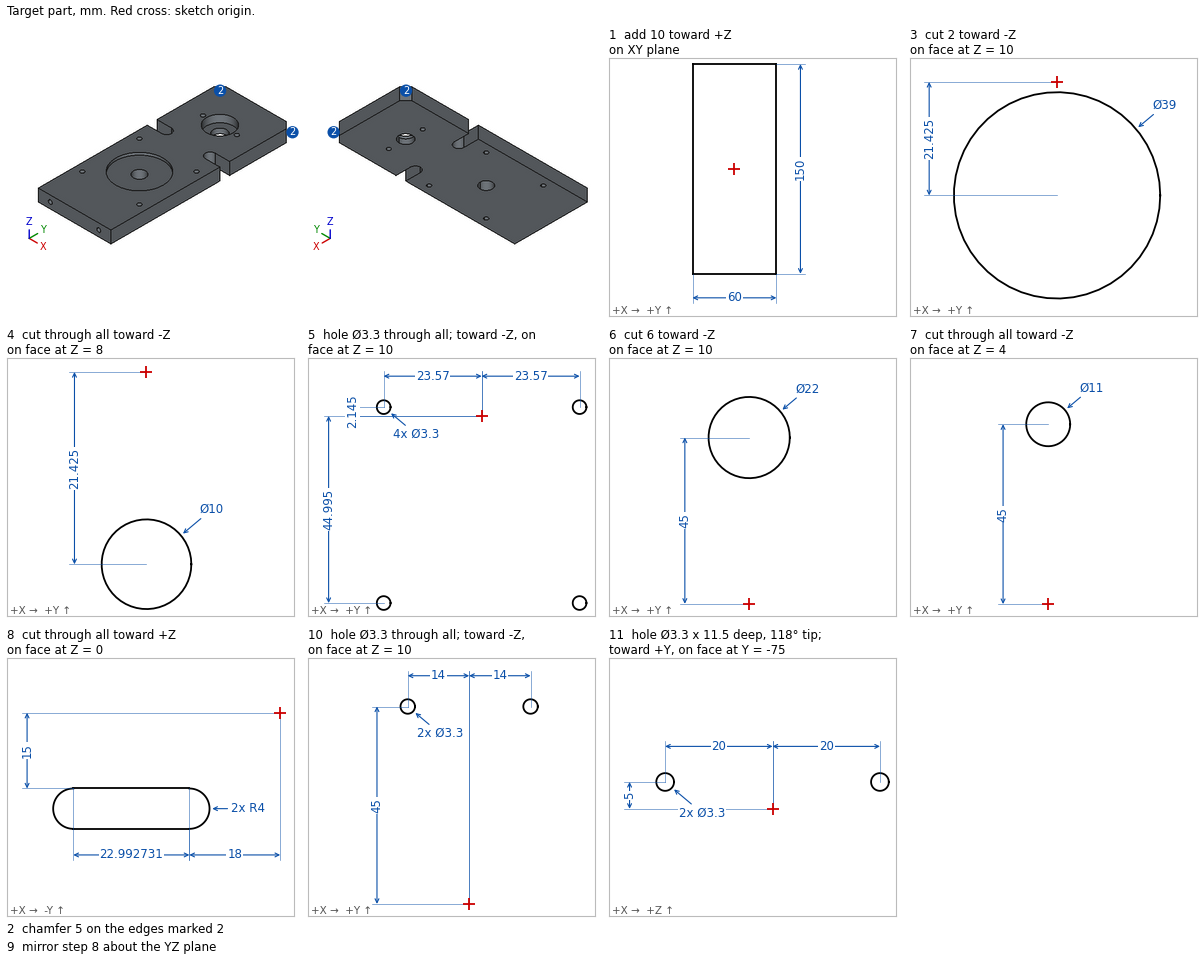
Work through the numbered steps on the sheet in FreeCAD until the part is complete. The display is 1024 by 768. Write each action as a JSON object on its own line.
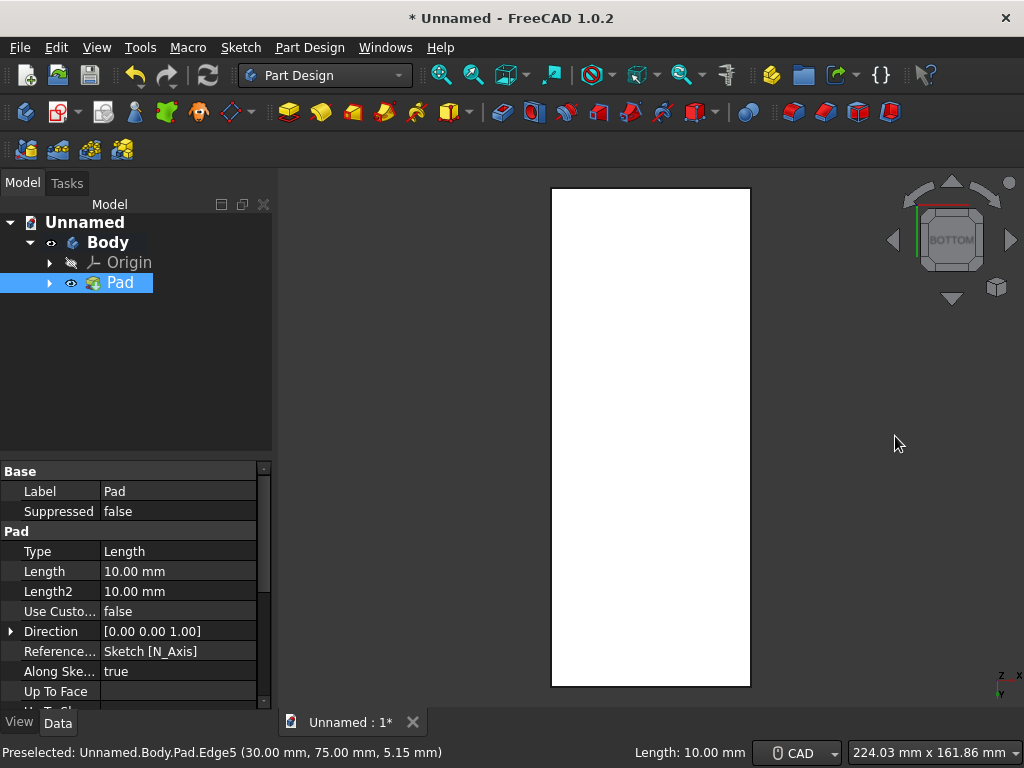
{"action": "key", "text": "4"}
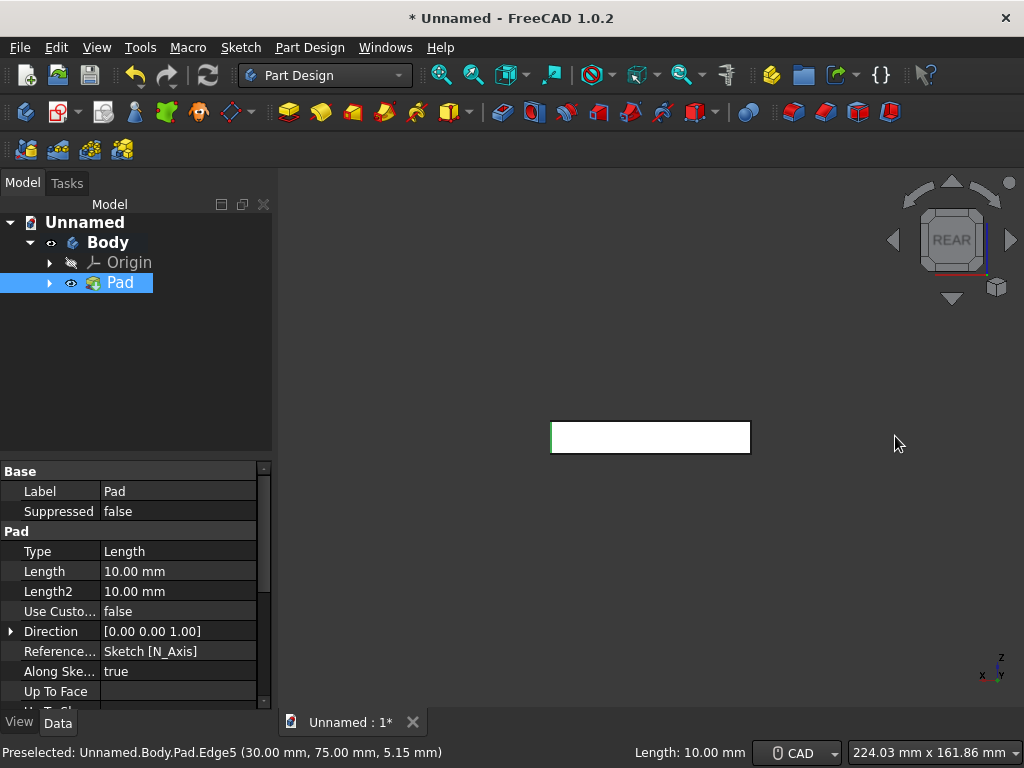
{"action": "left_click", "coordinate": [442, 76]}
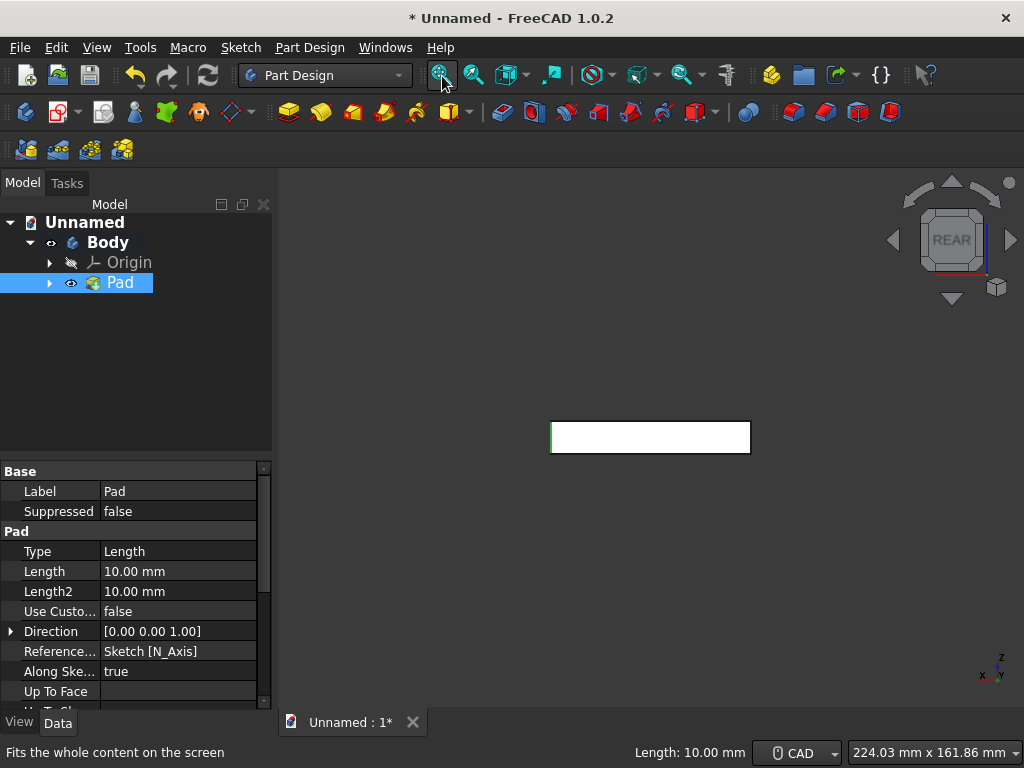
{"action": "left_click", "coordinate": [751, 437], "text": "ctrl"}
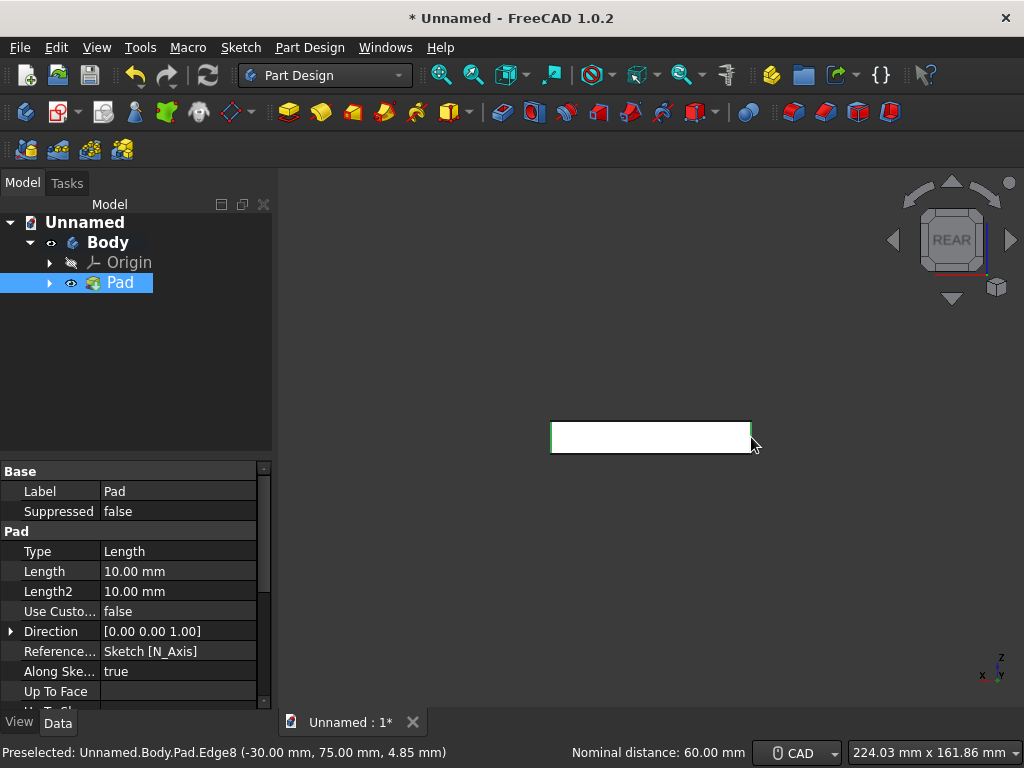
{"action": "left_click", "coordinate": [826, 112]}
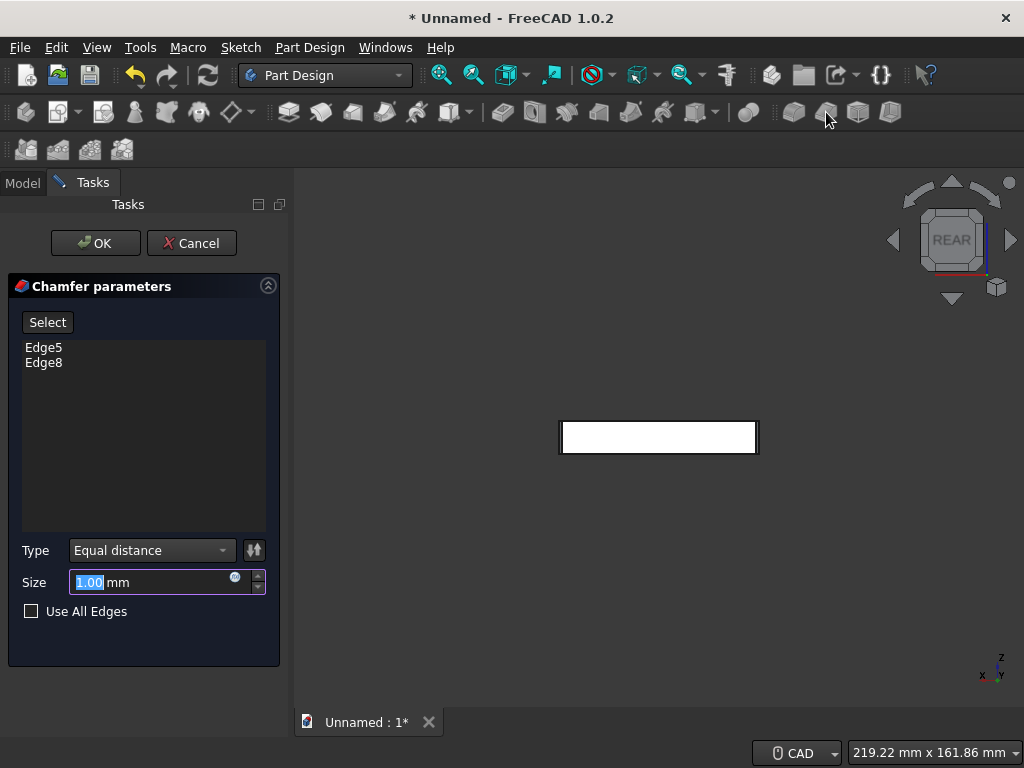
{"action": "type", "text": "5"}
{"action": "key", "text": "Tab"}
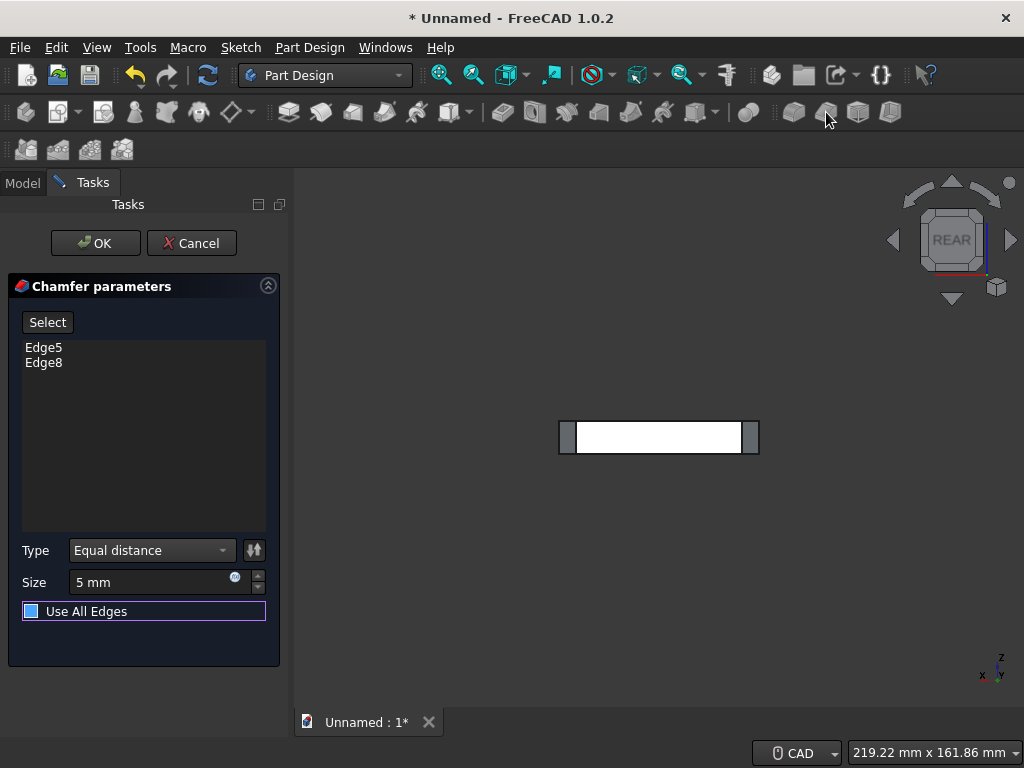
{"action": "left_click", "coordinate": [96, 243]}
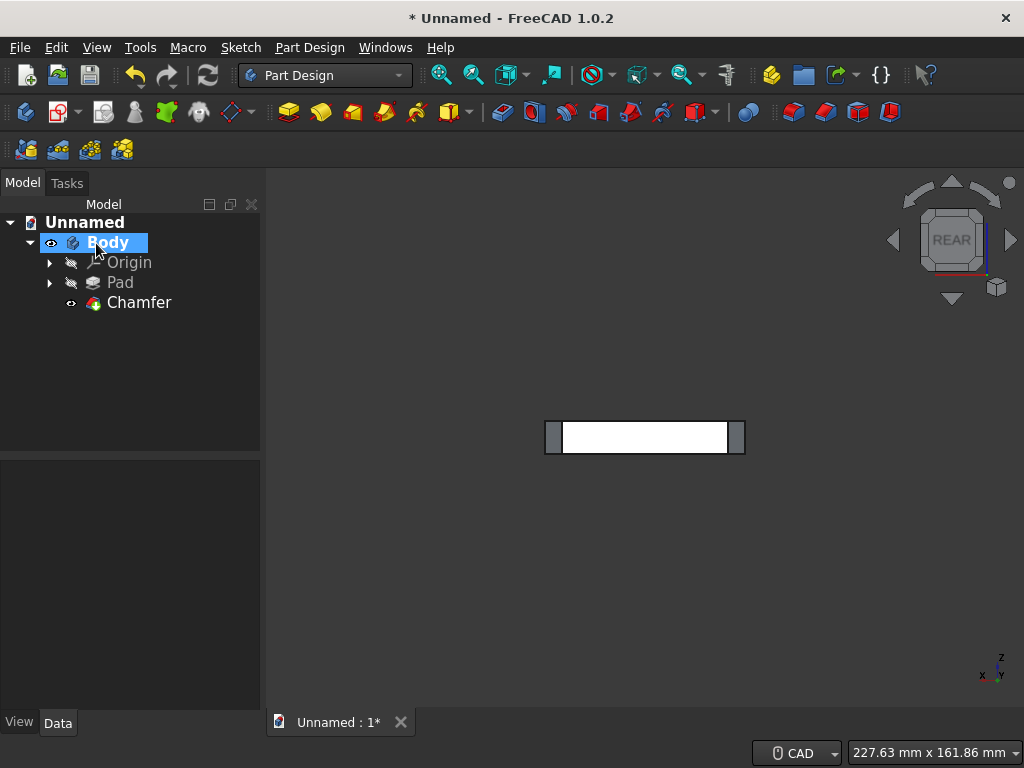
{"action": "left_click", "coordinate": [442, 76]}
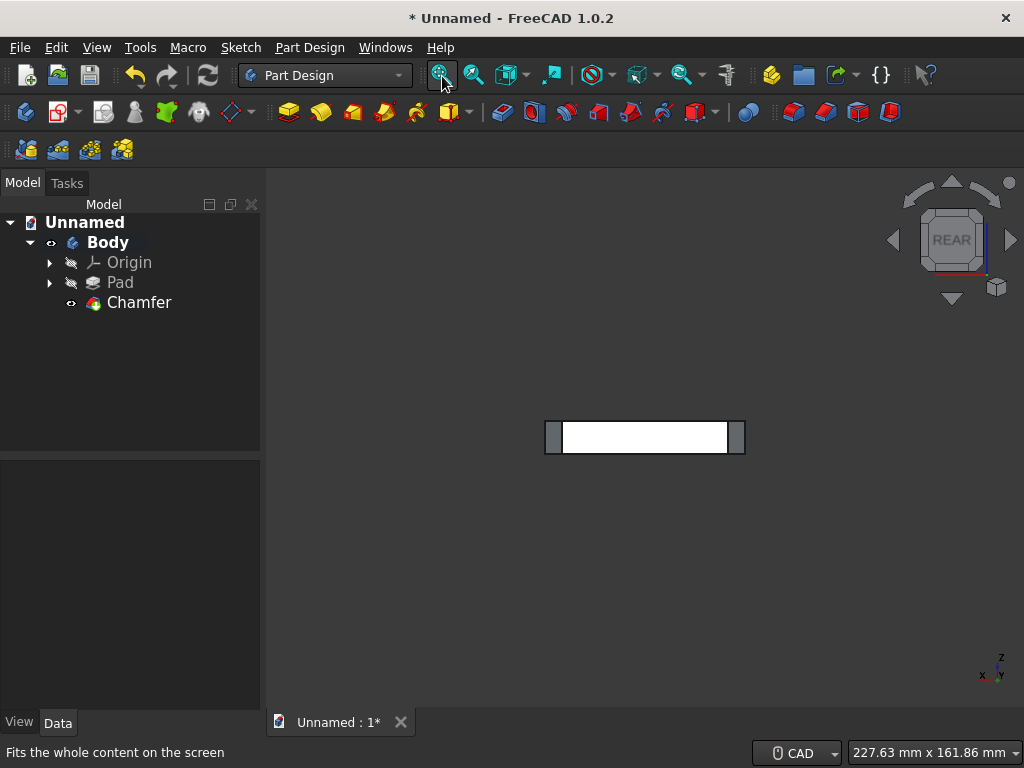
{"action": "key", "text": "0"}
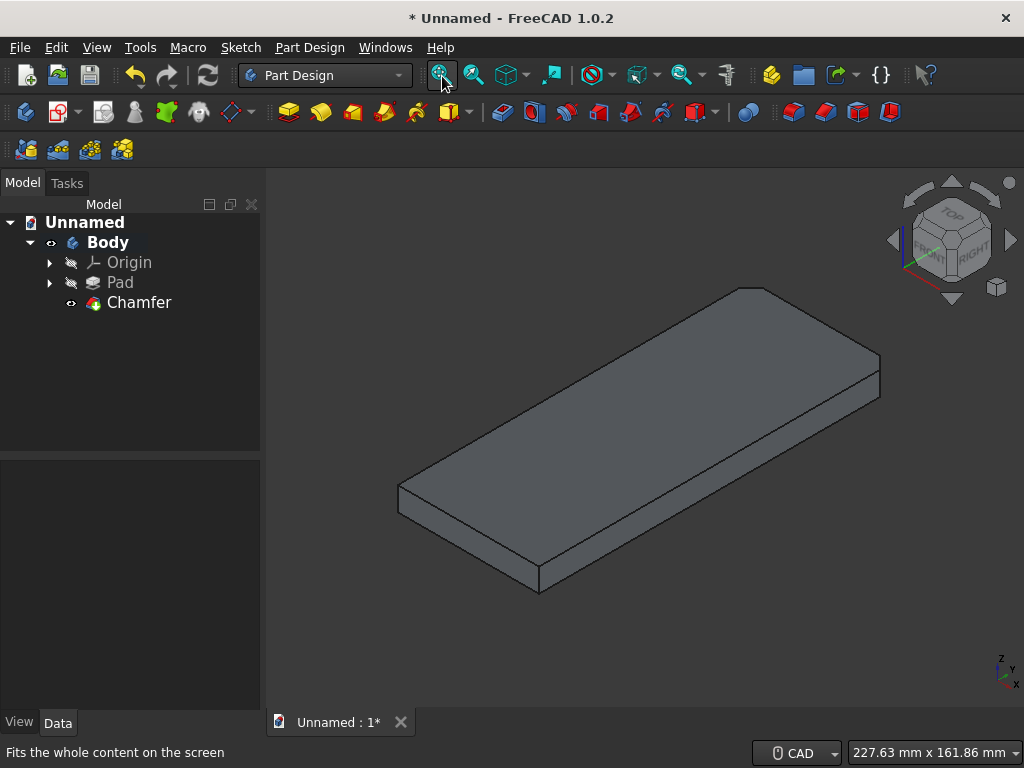
{"action": "left_click", "coordinate": [746, 365]}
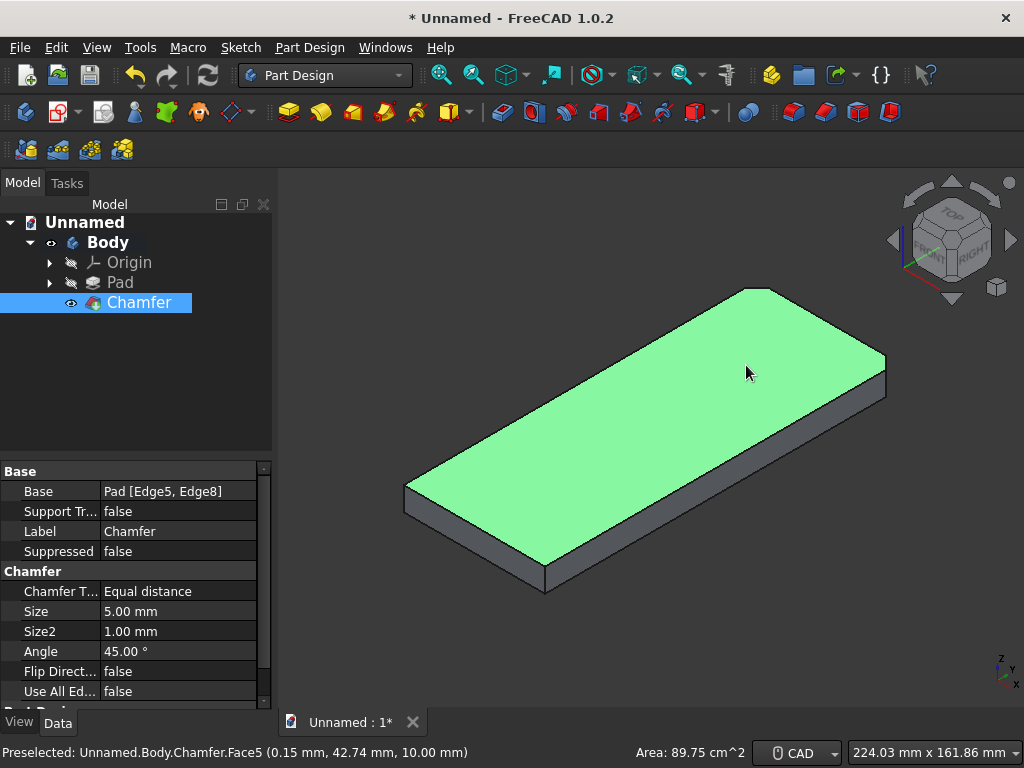
{"action": "left_click", "coordinate": [58, 112]}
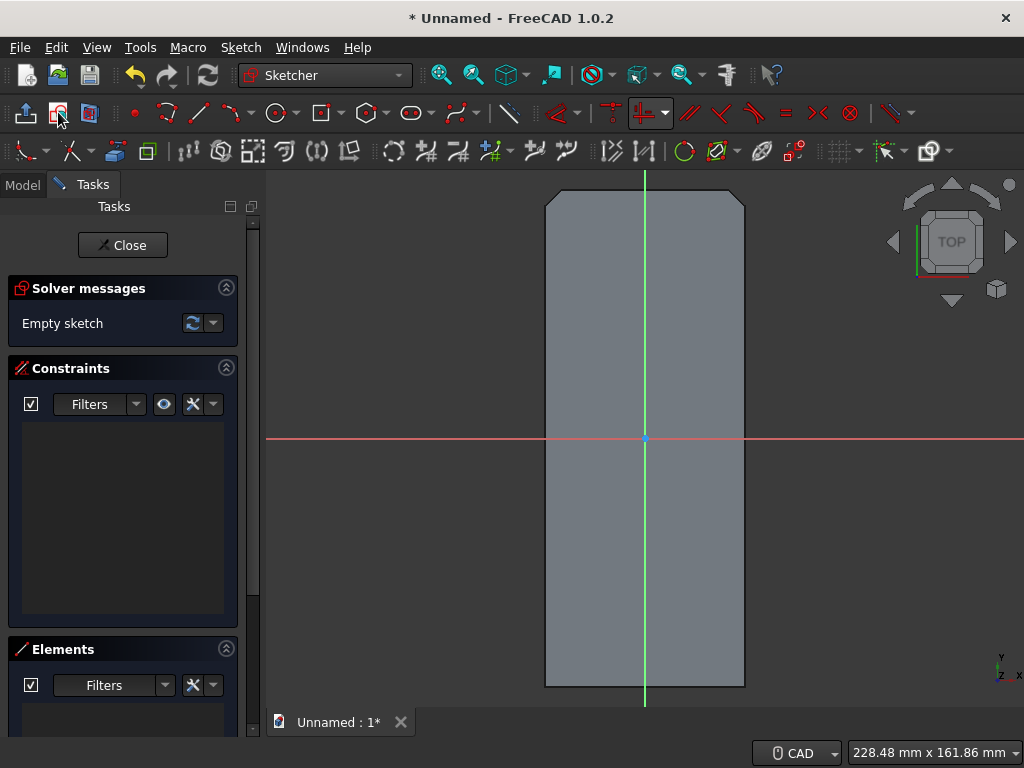
{"action": "scroll", "coordinate": [685, 546], "scroll_direction": "up", "scroll_amount": 5}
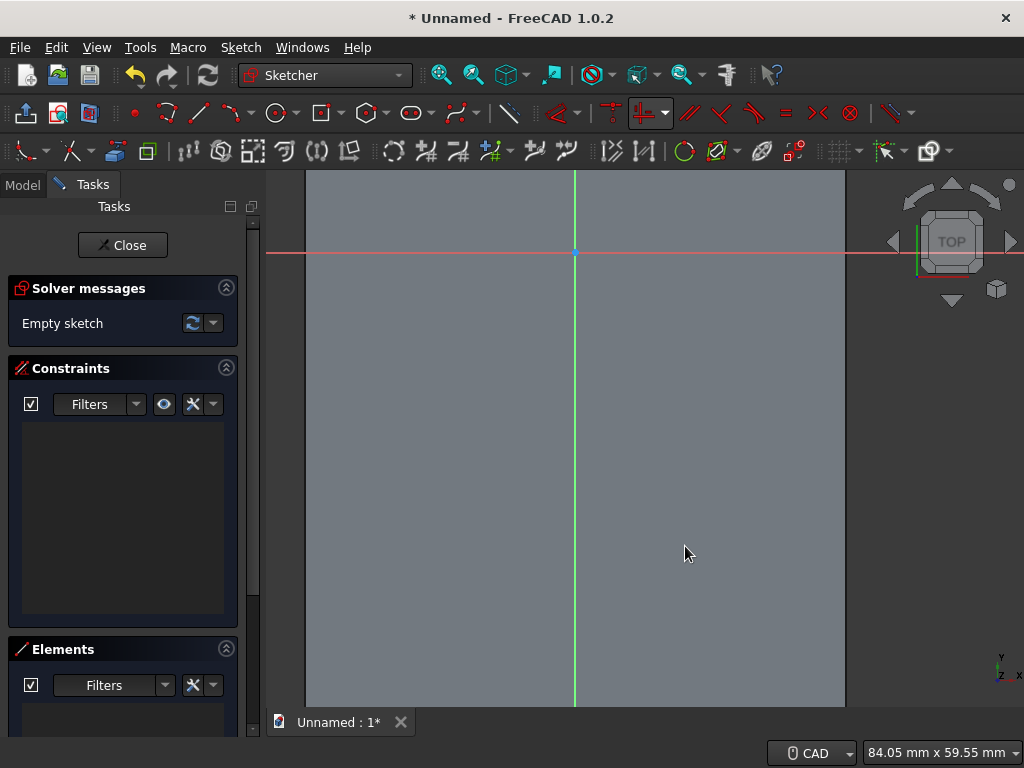
{"action": "left_click", "coordinate": [276, 114]}